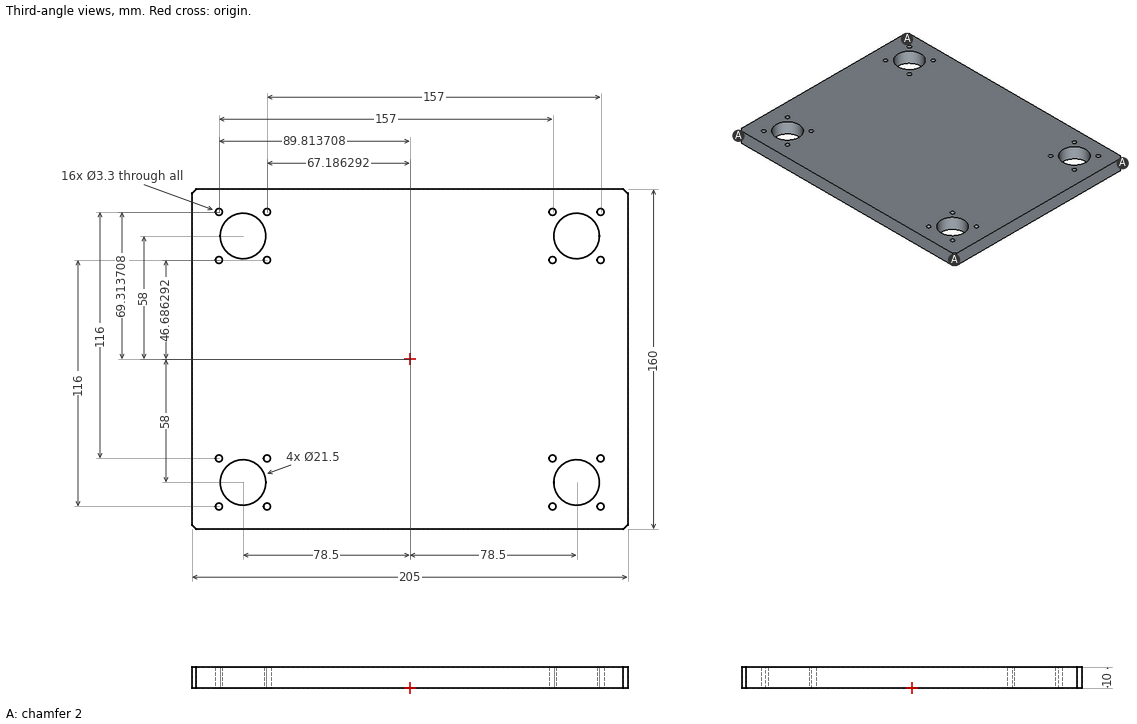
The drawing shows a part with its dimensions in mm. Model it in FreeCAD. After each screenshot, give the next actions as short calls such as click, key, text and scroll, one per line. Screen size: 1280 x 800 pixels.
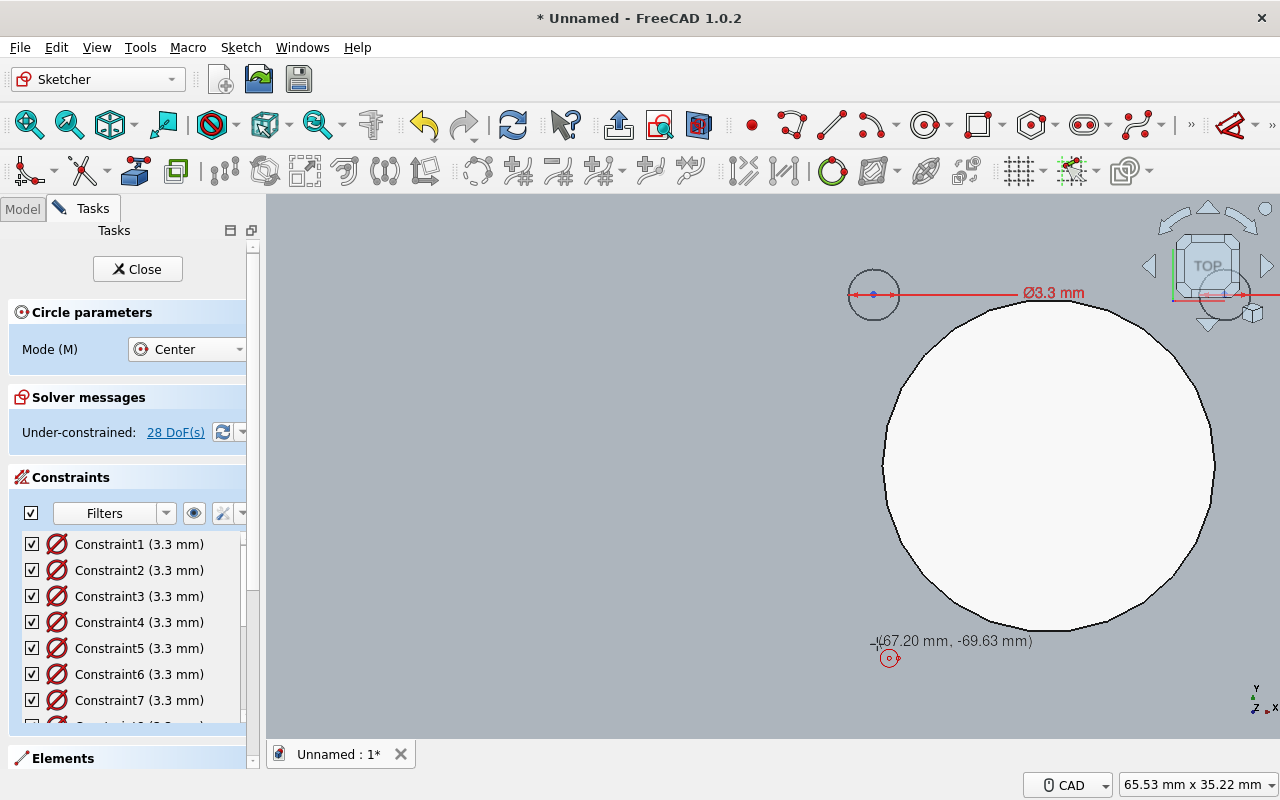
scroll(877, 644, down, 9)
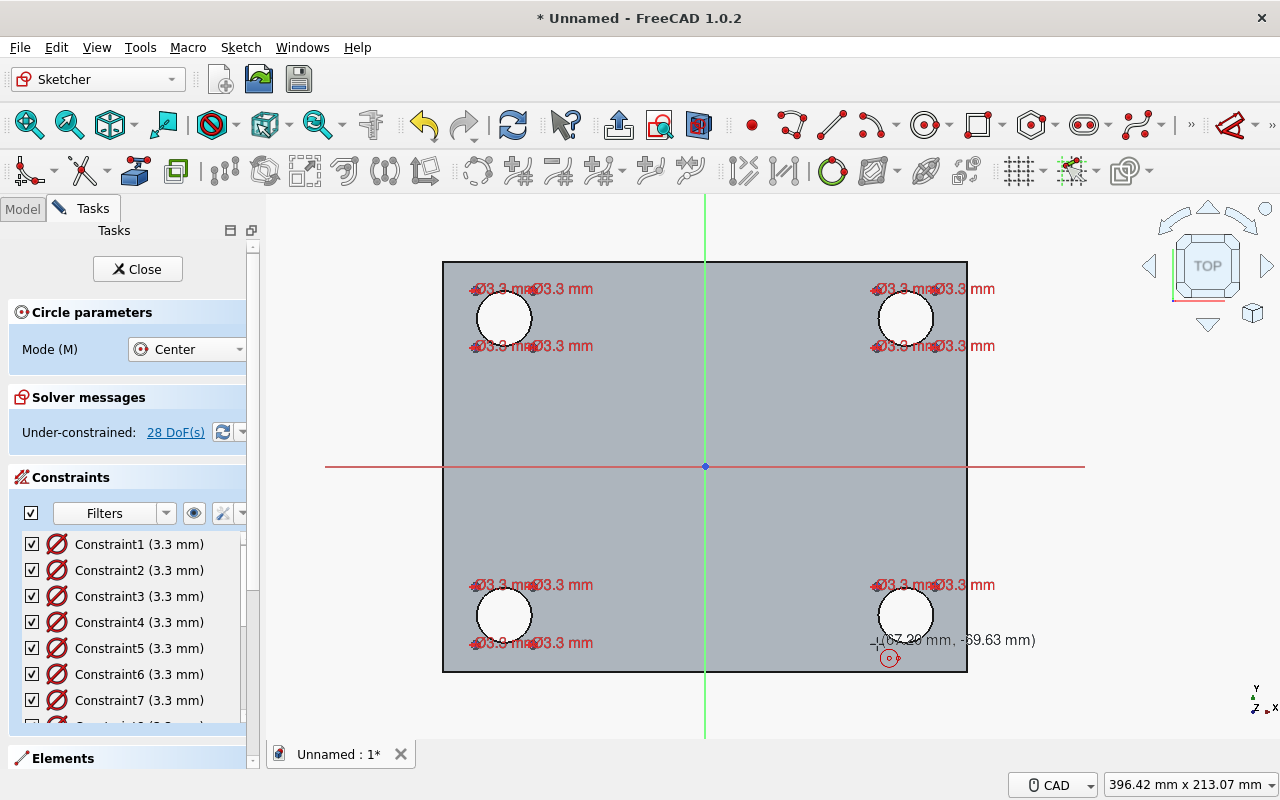
click(877, 644)
move(880, 641)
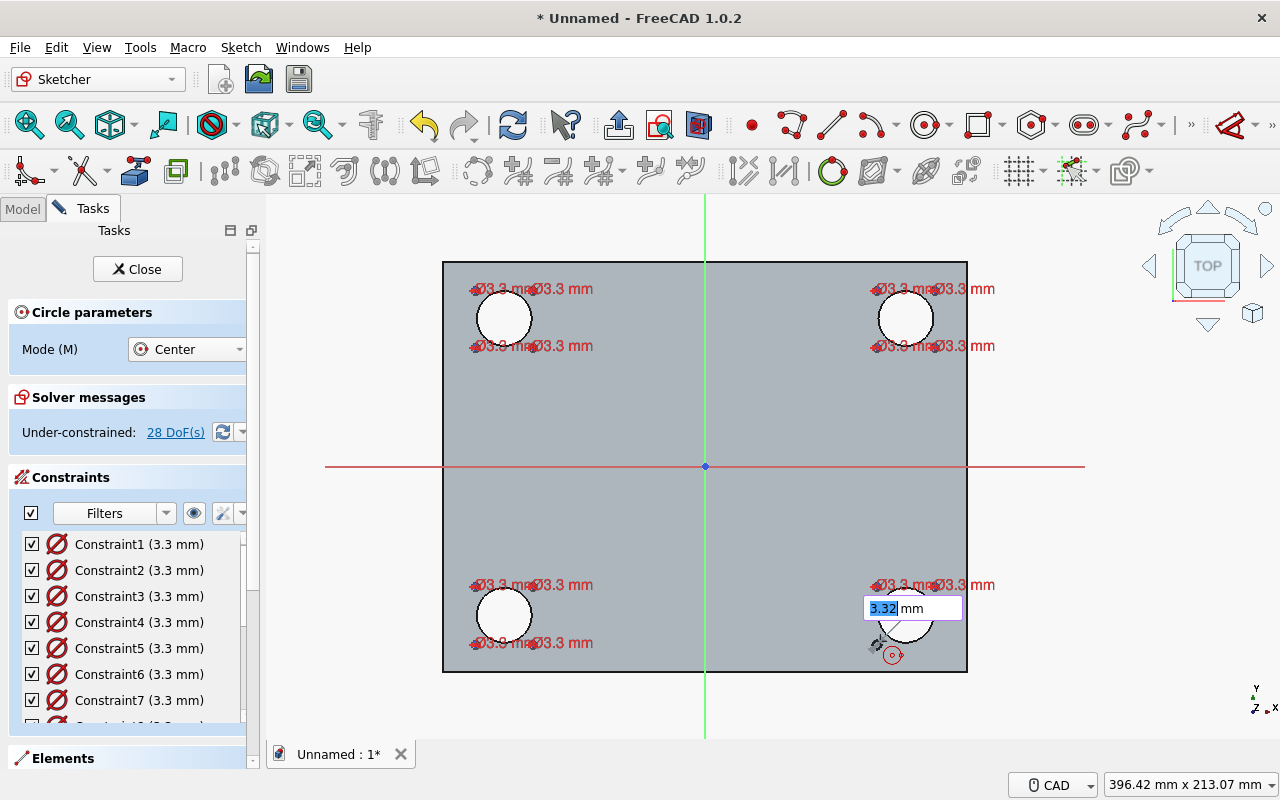
text(3.3)
key(Return)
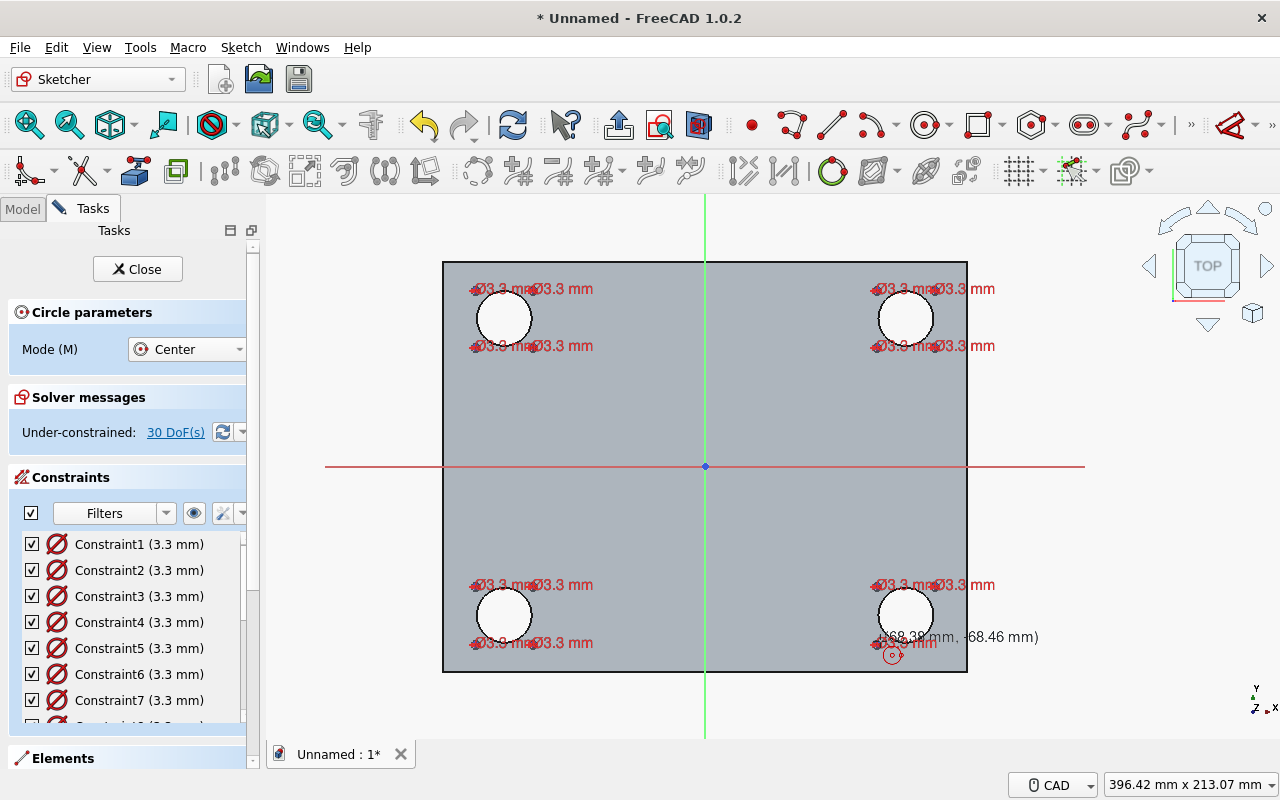
scroll(935, 644, up, 9)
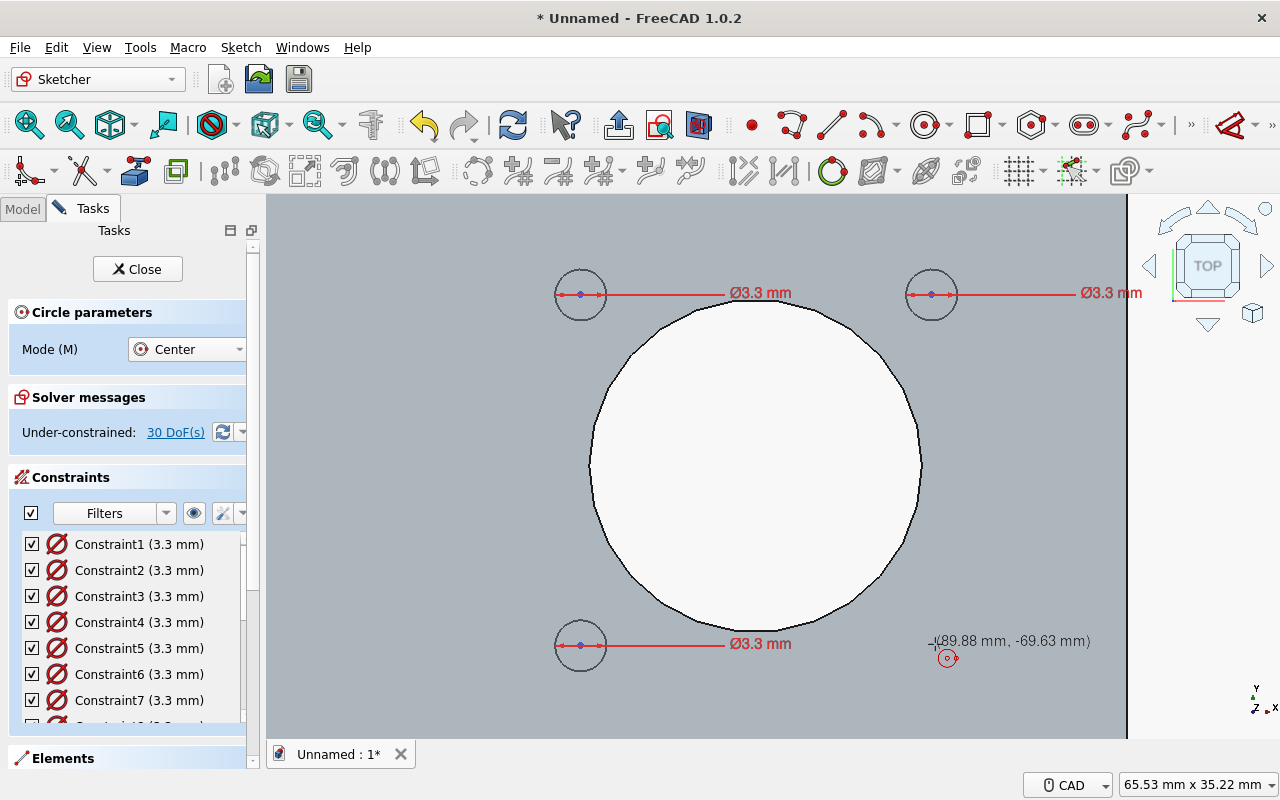
scroll(935, 644, down, 9)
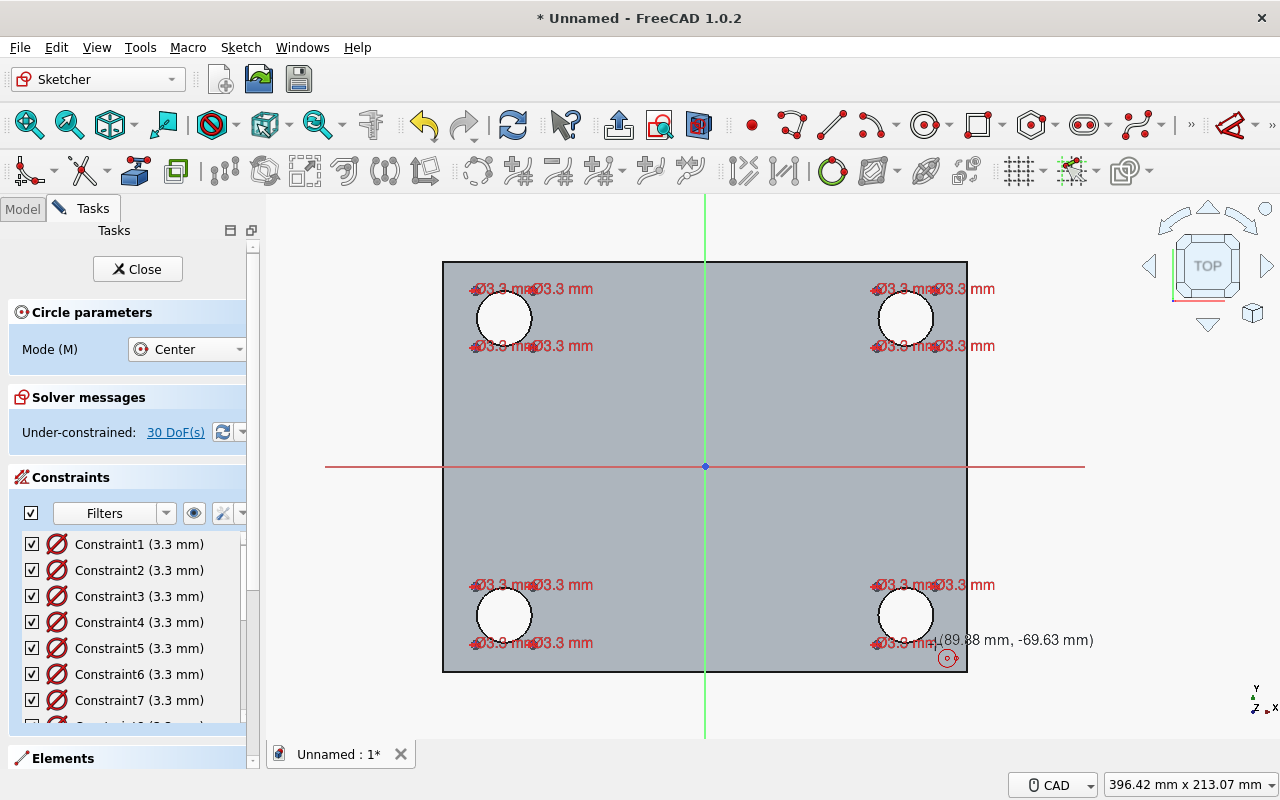
click(935, 644)
move(938, 641)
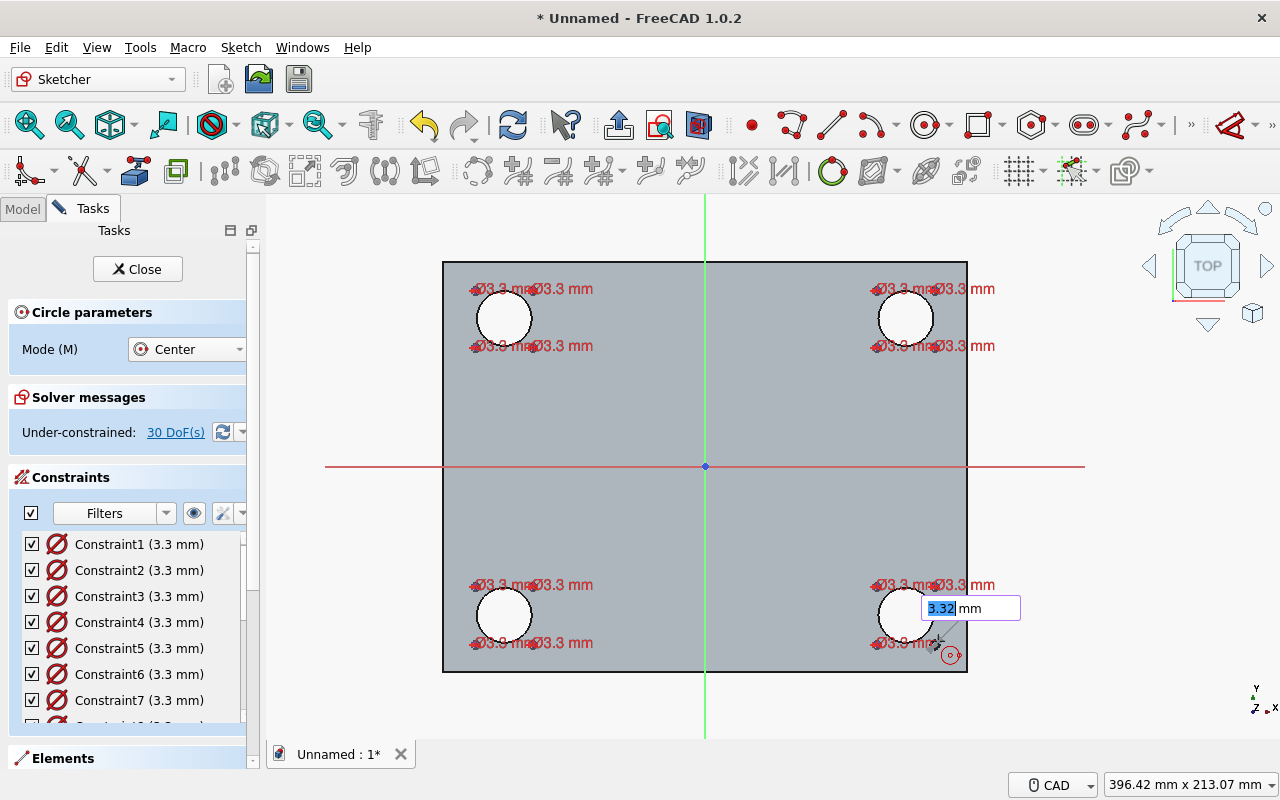
text(3.3)
key(Return)
key(Escape)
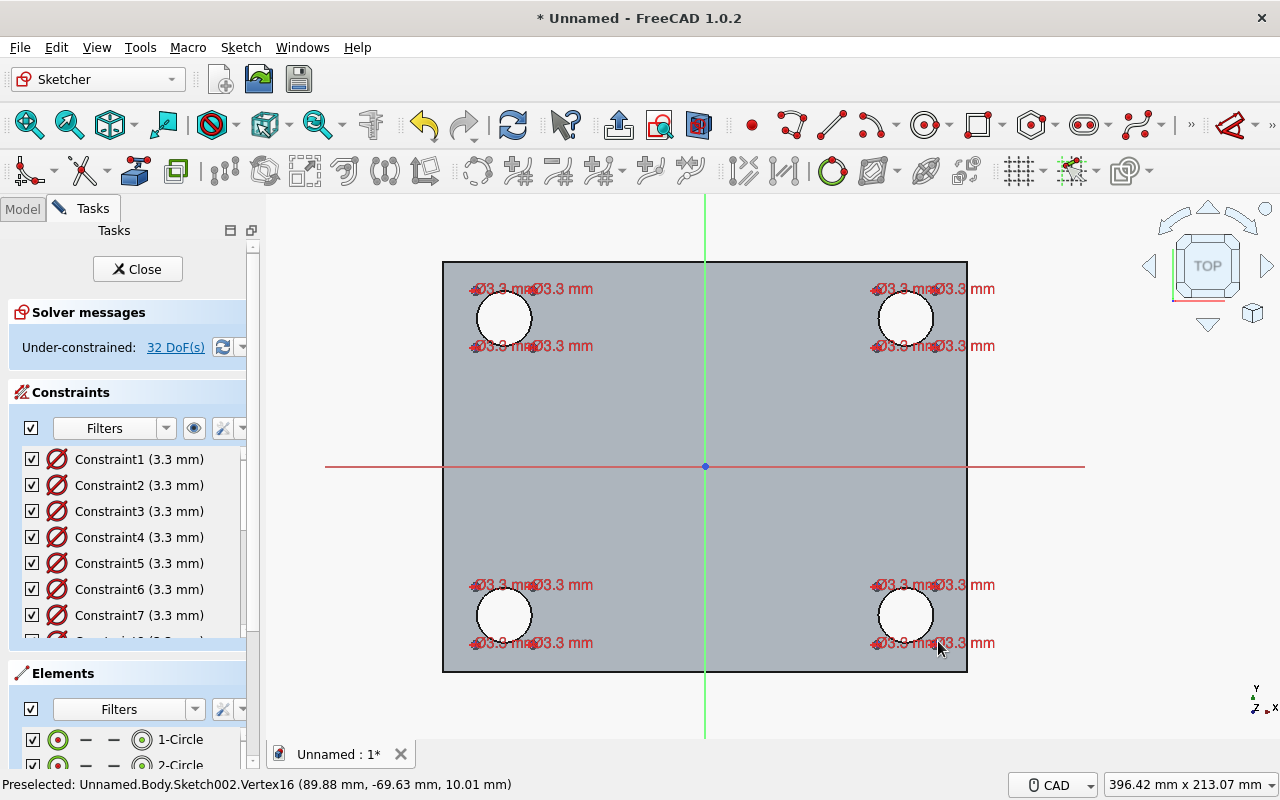
click(476, 291)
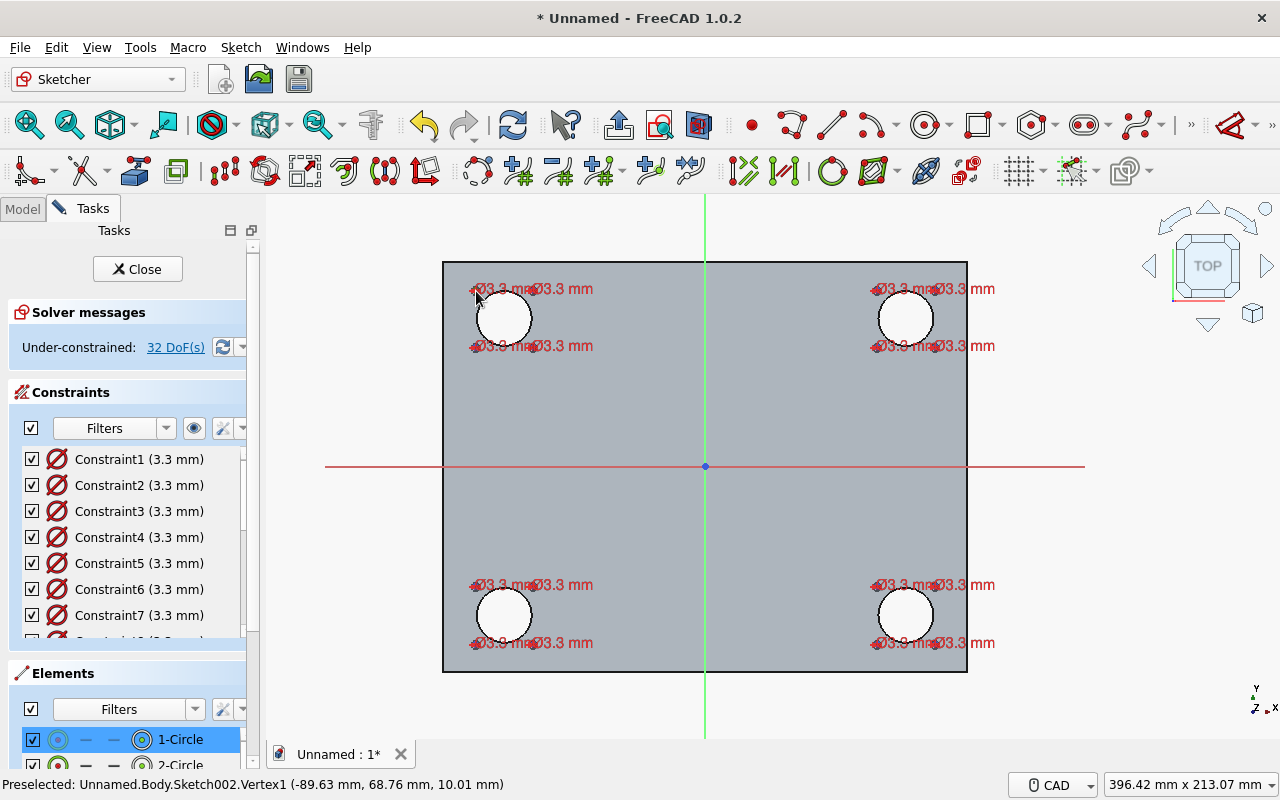
click(533, 291)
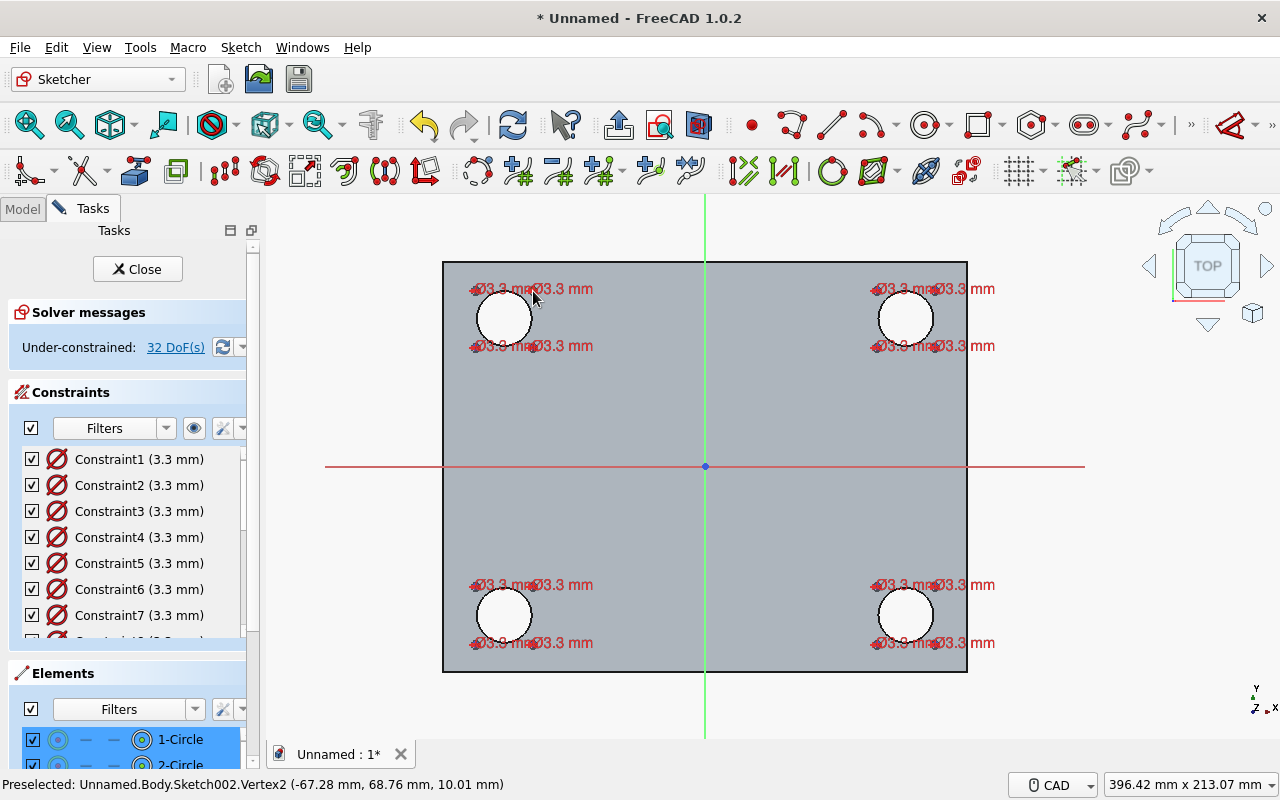
key(h)